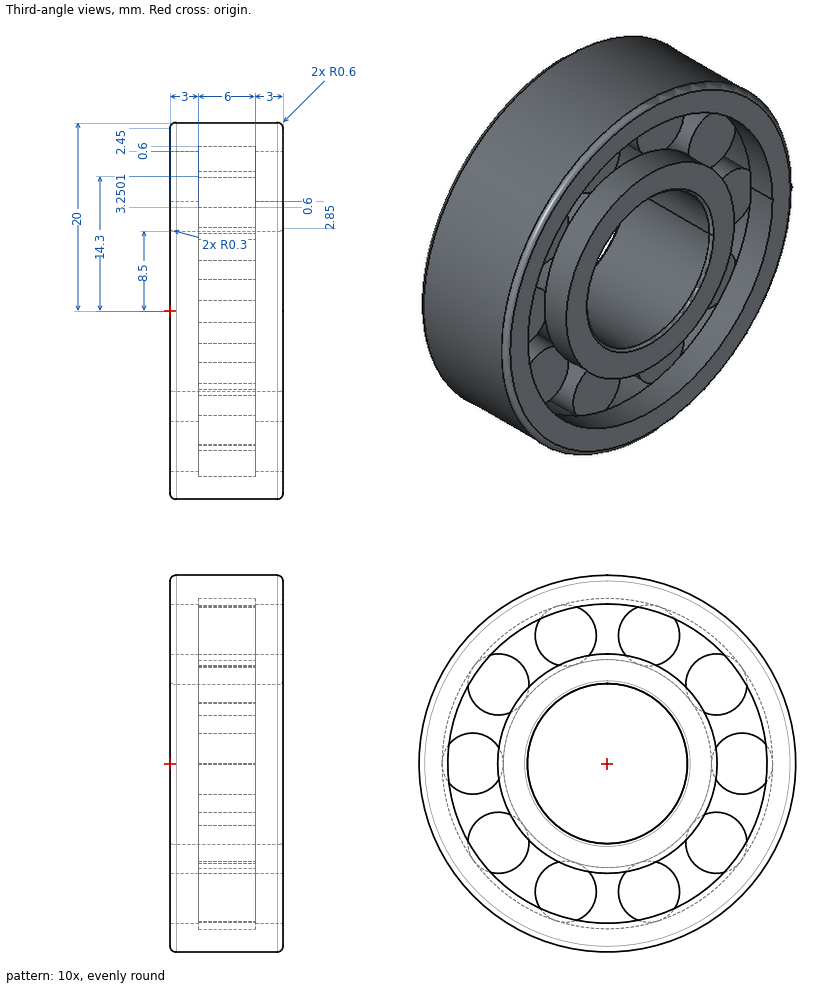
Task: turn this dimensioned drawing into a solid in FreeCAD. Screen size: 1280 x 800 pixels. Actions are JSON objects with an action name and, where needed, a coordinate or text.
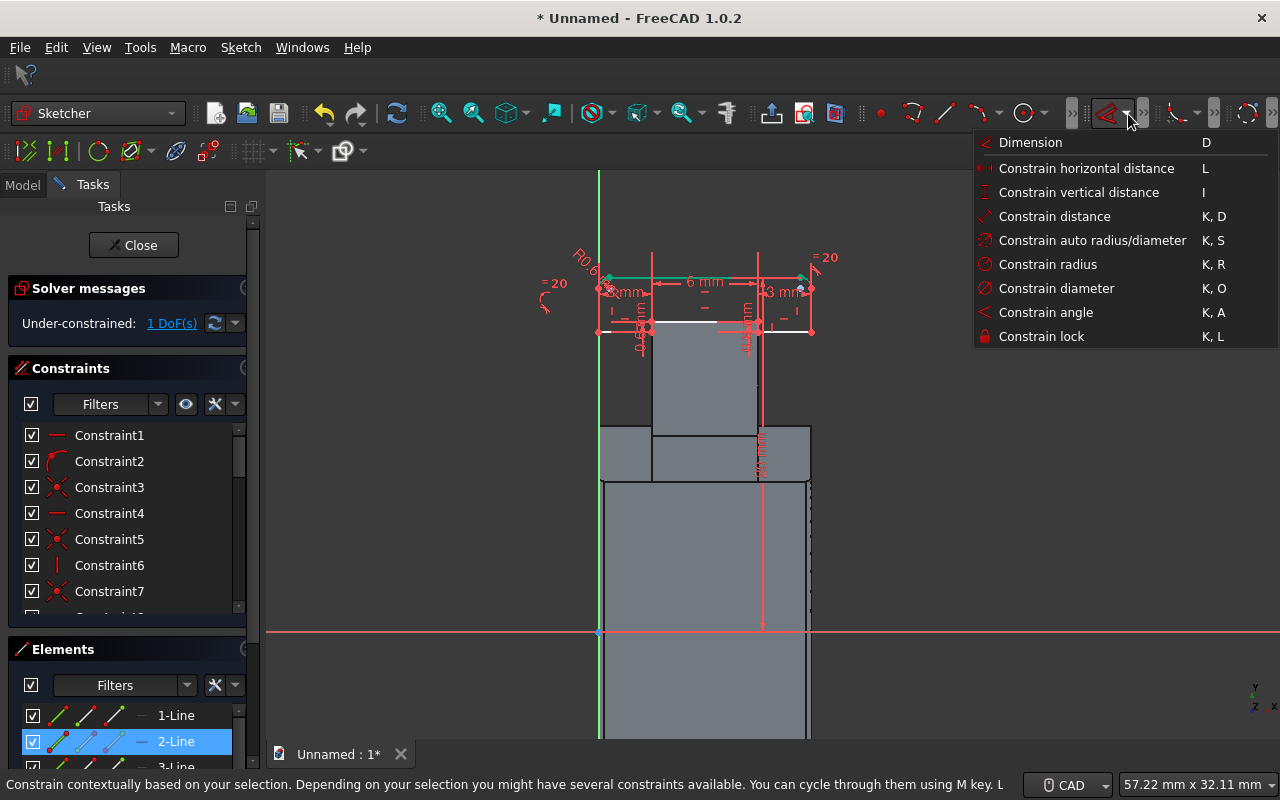
{"action": "left_click", "coordinate": [1126, 192]}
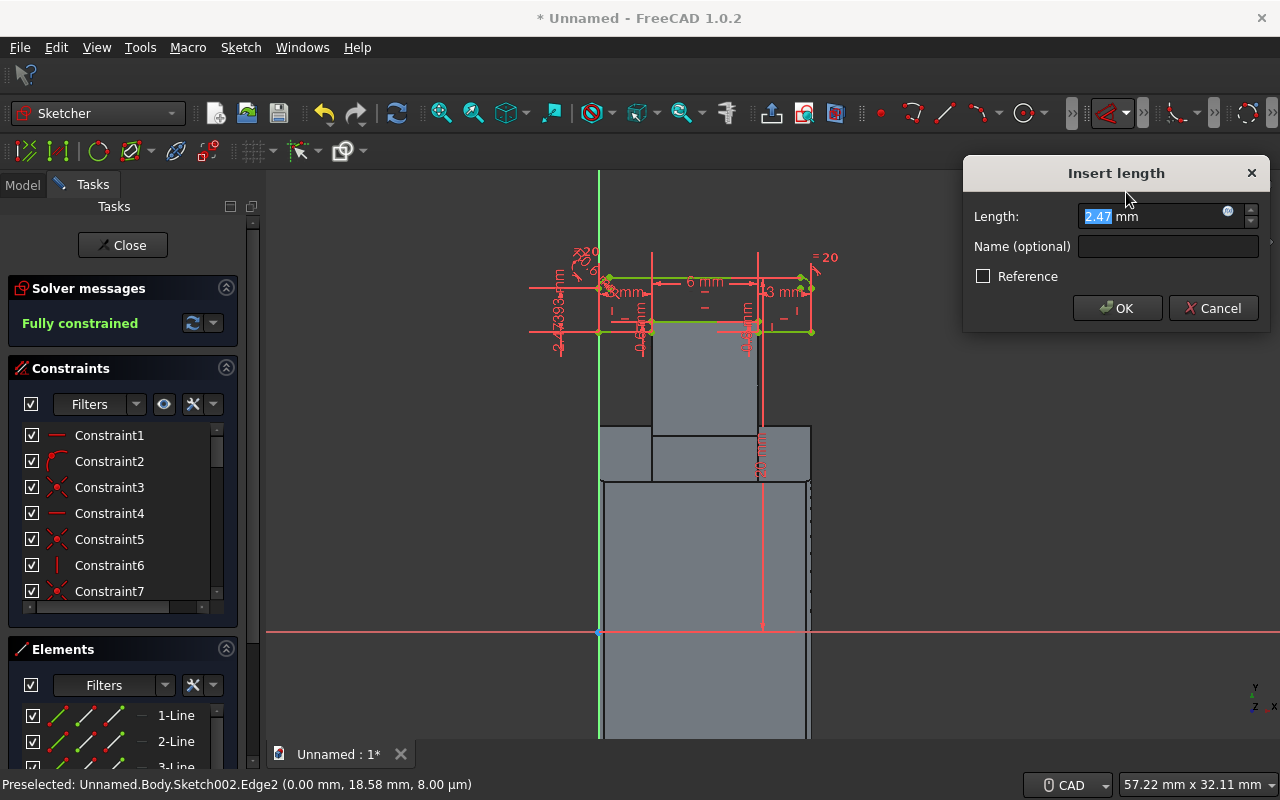
{"action": "type", "text": "2.45"}
{"action": "key", "text": "Return"}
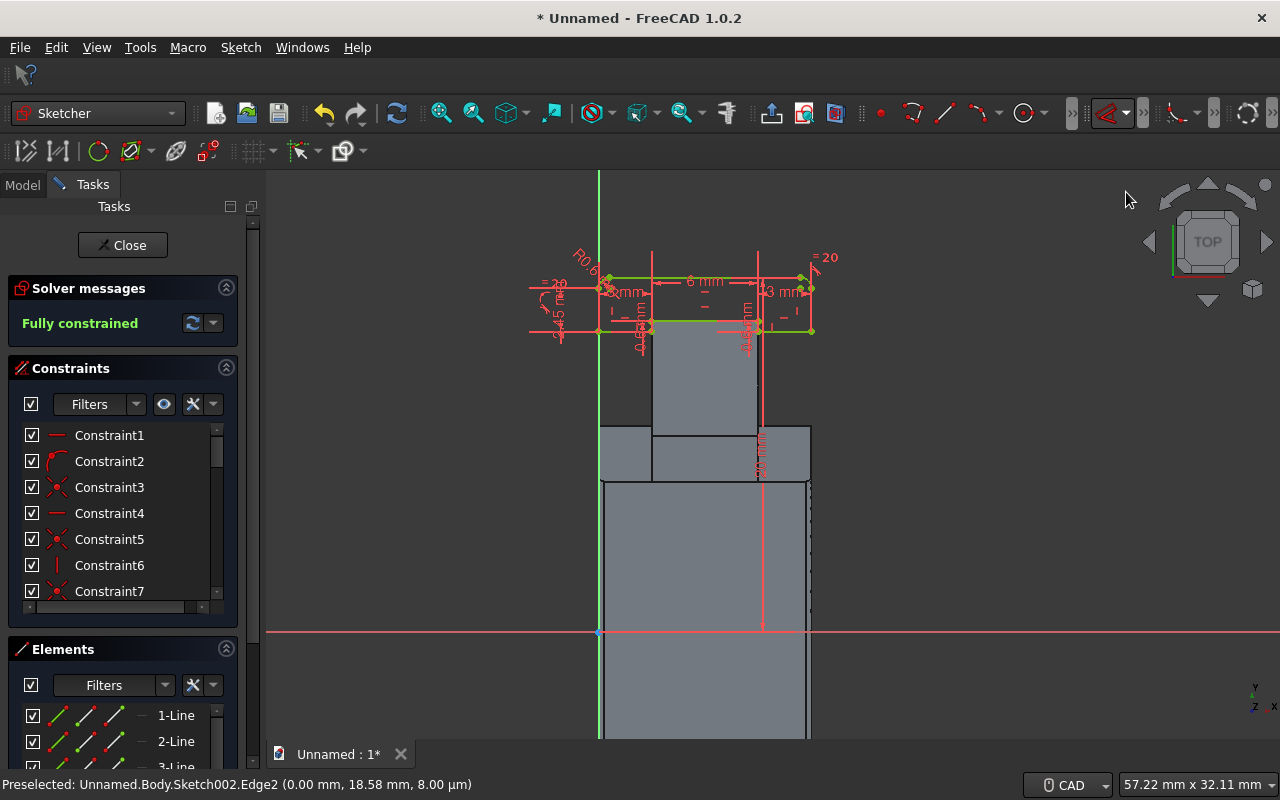
{"action": "left_click", "coordinate": [123, 245]}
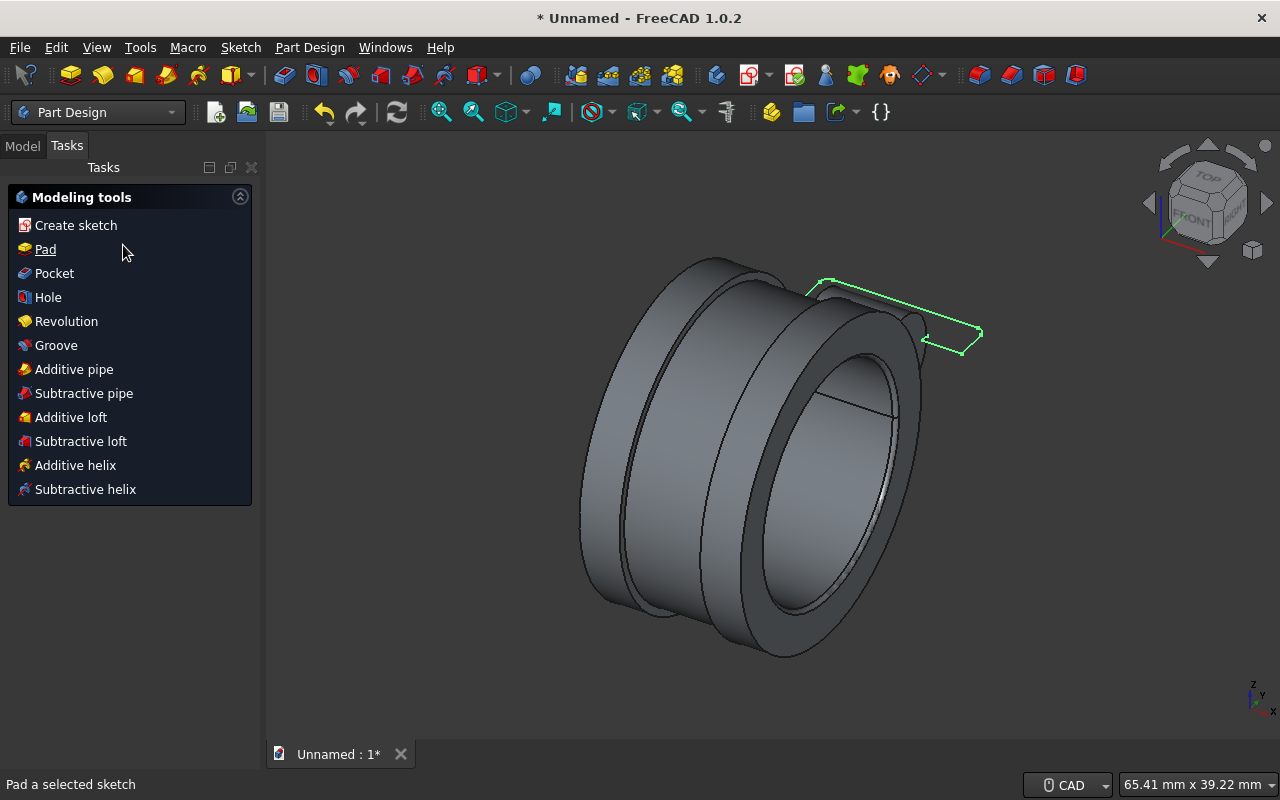
{"action": "left_click", "coordinate": [104, 76]}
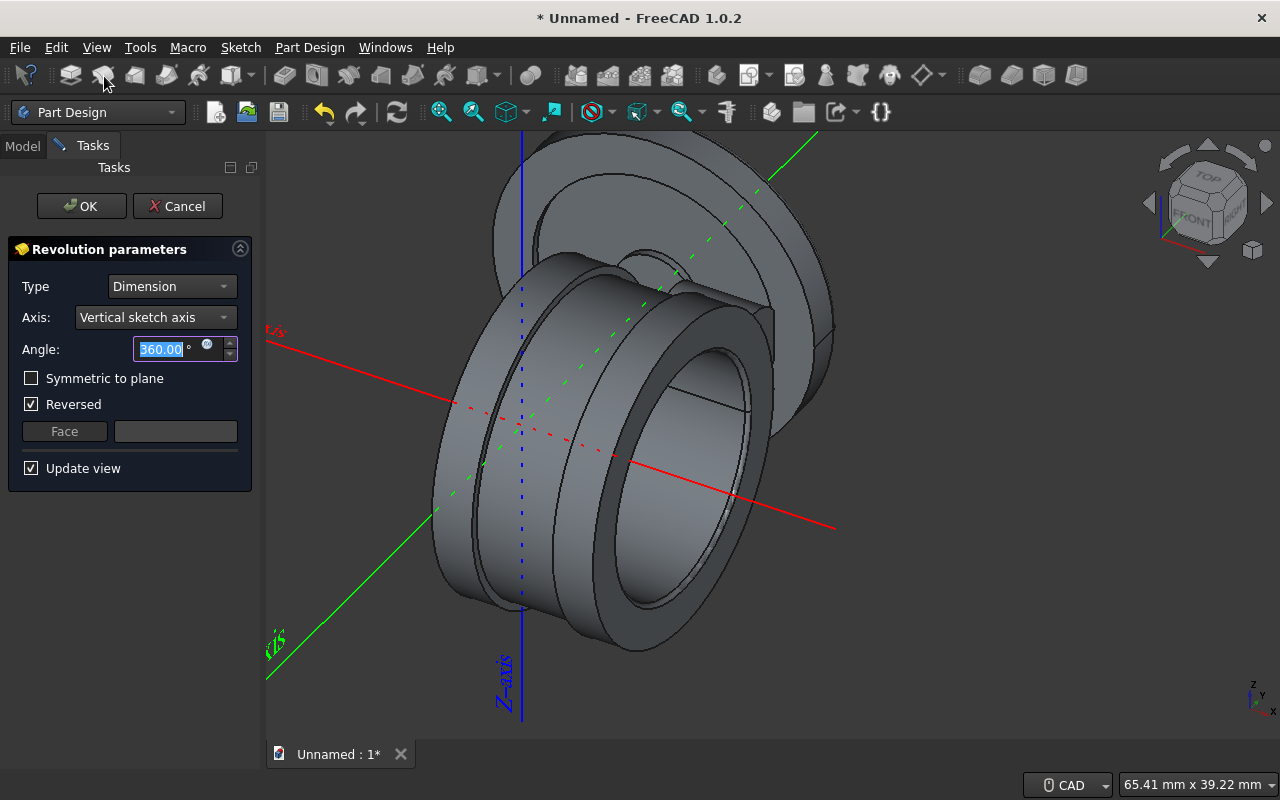
{"action": "left_click", "coordinate": [156, 318]}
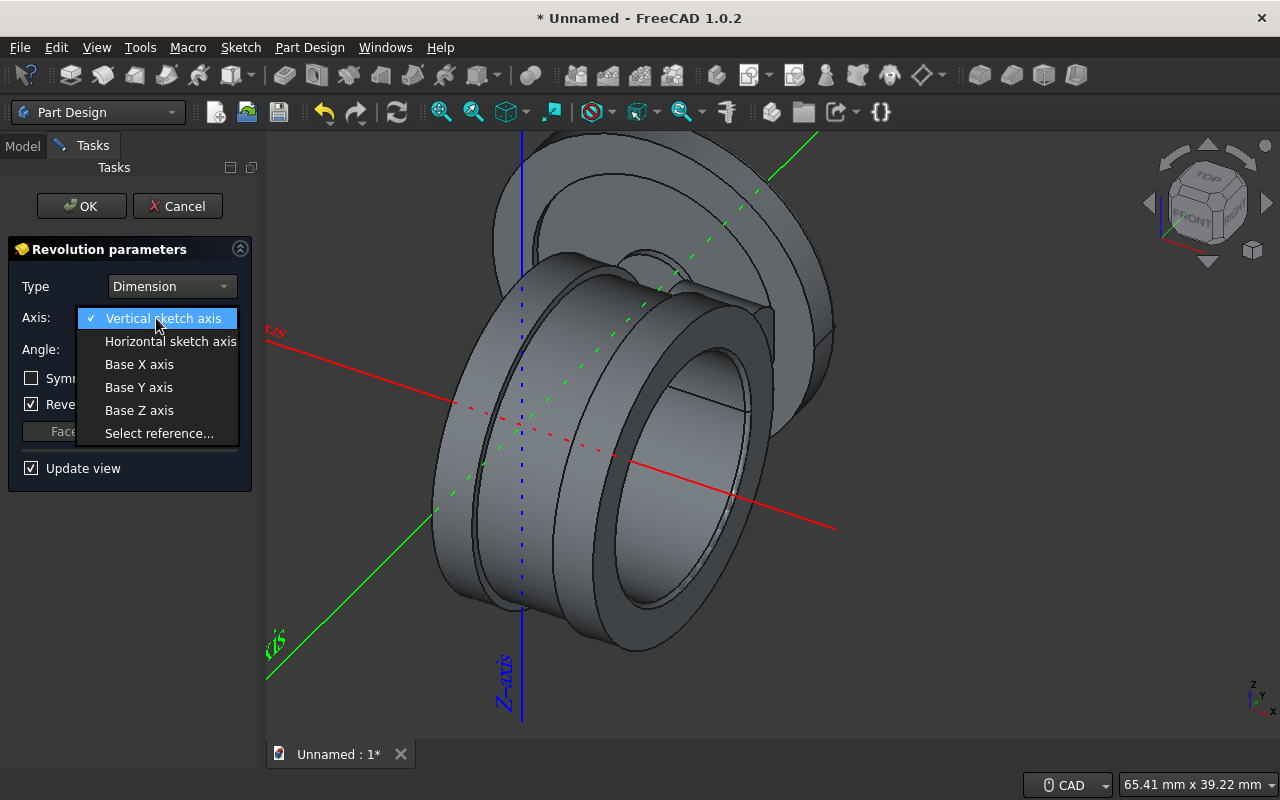
{"action": "left_click", "coordinate": [156, 342]}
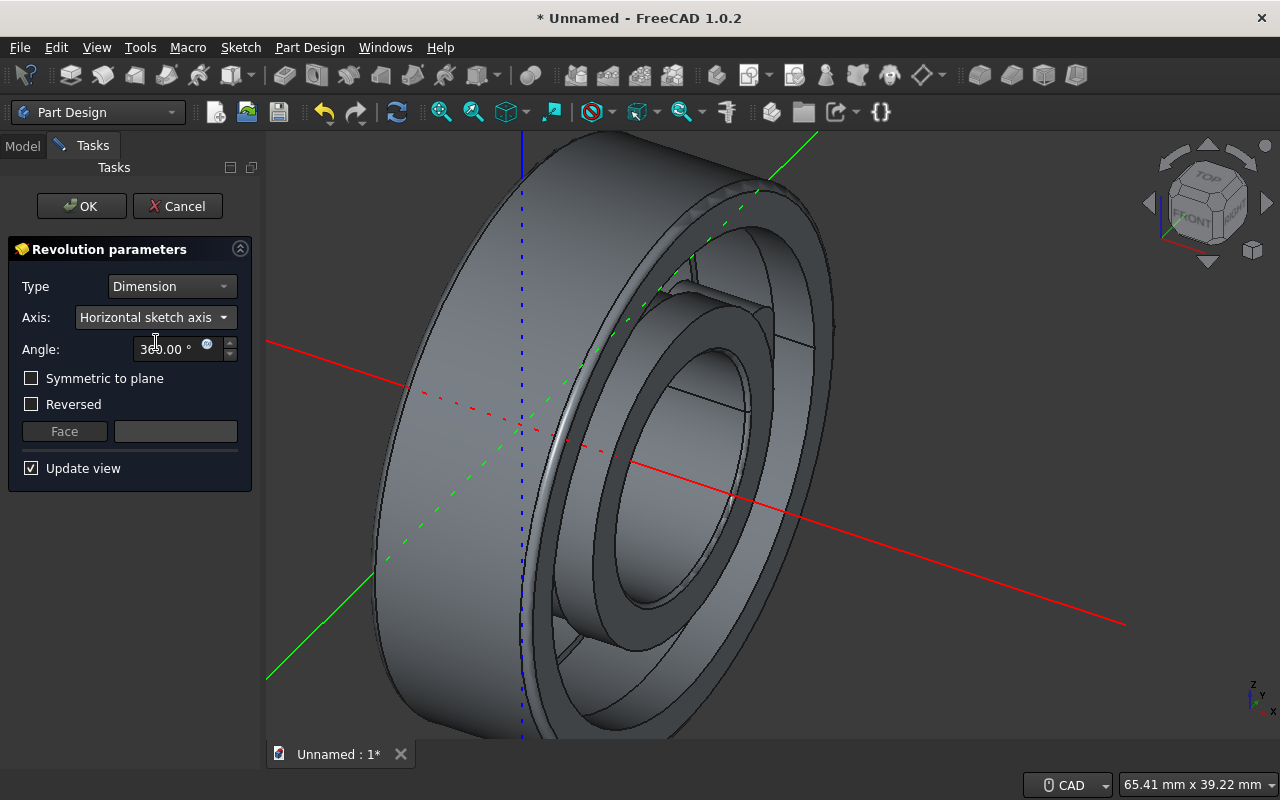
{"action": "left_click", "coordinate": [82, 206]}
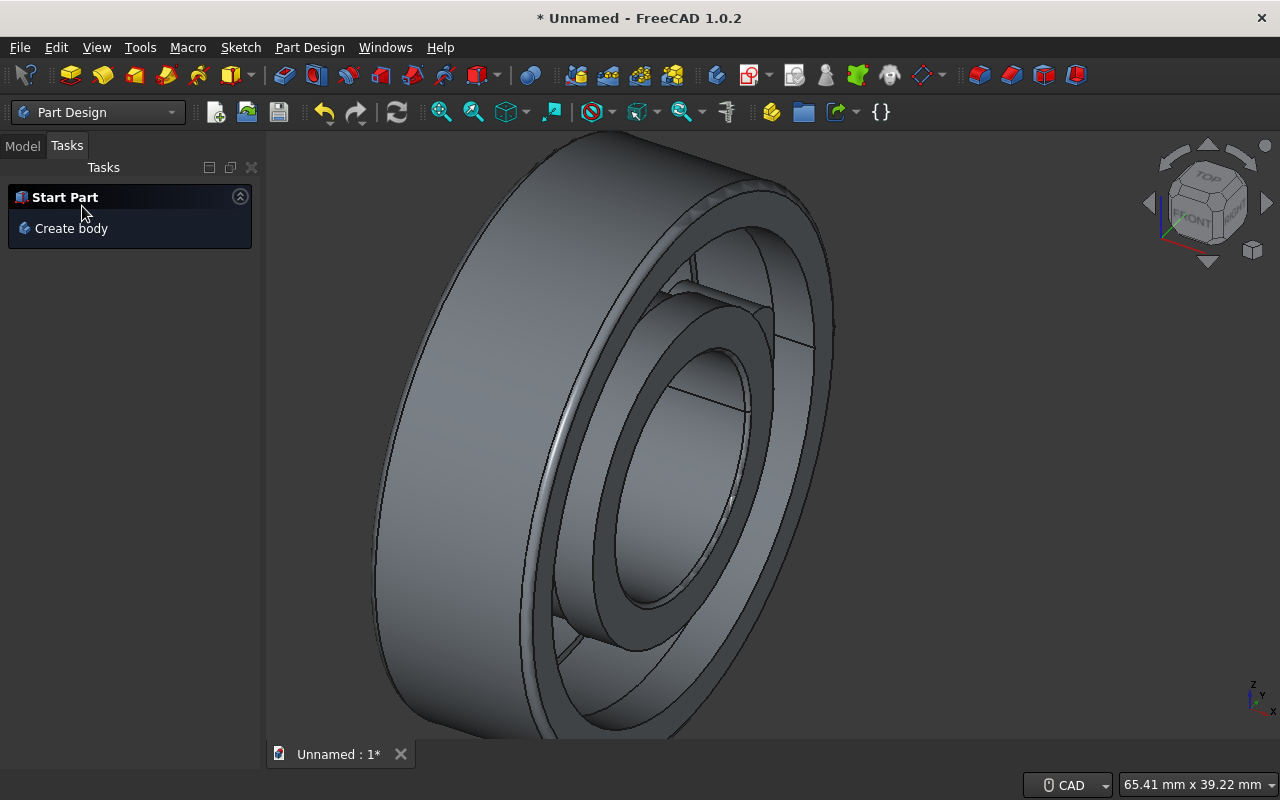
{"action": "left_click", "coordinate": [442, 112]}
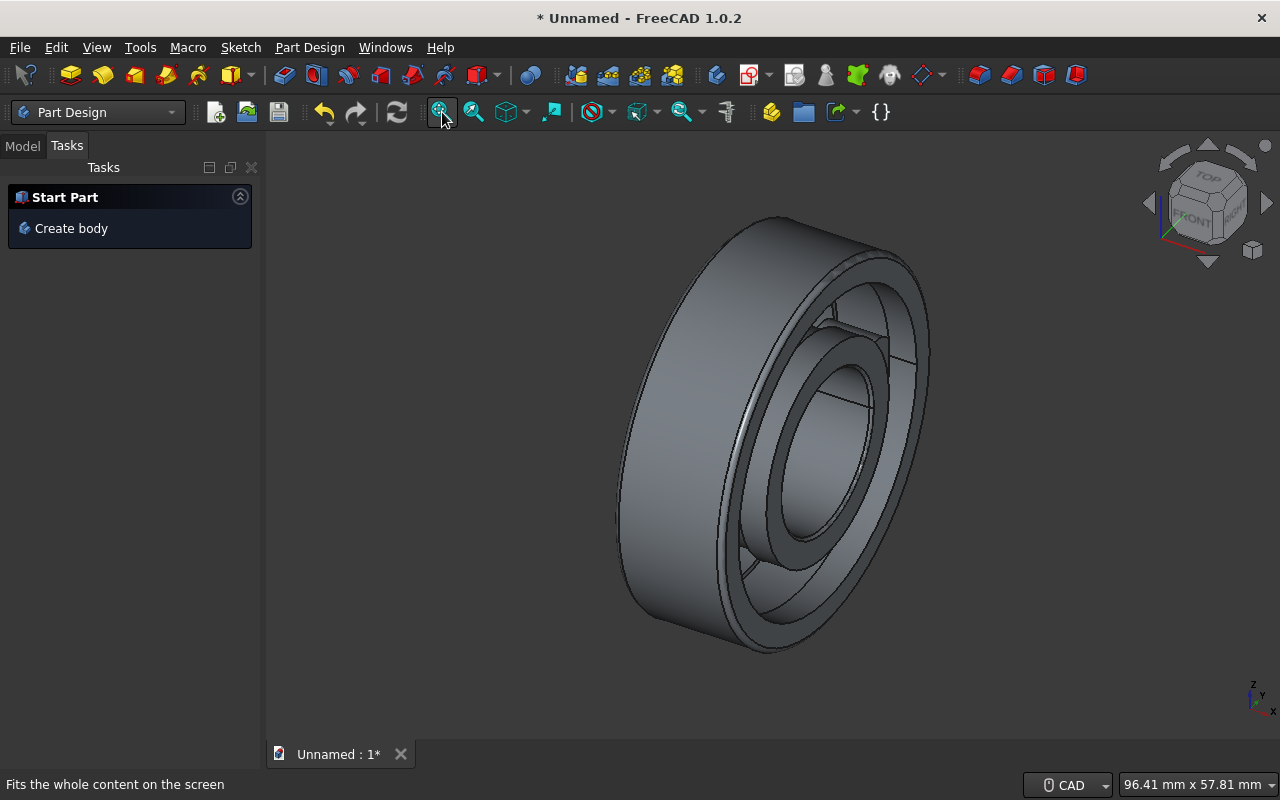
{"action": "left_click", "coordinate": [23, 145]}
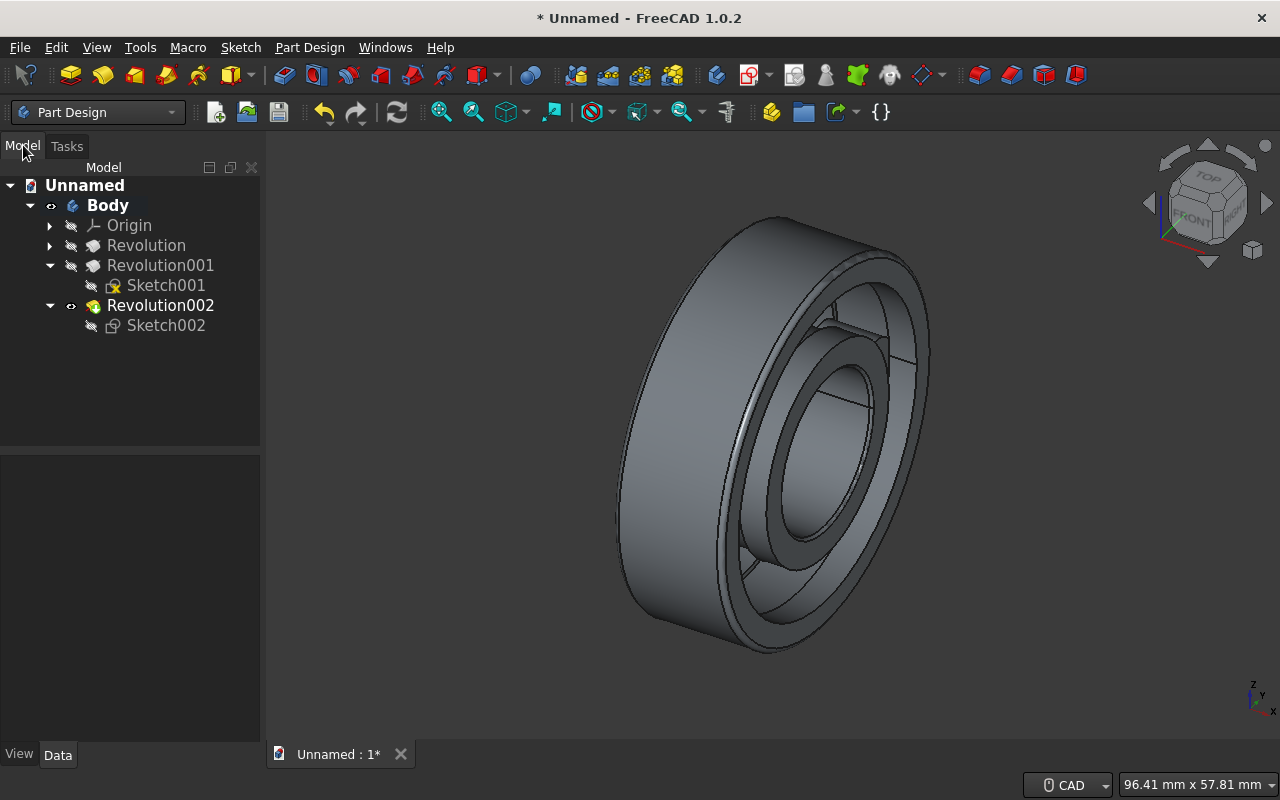
{"action": "left_click", "coordinate": [116, 266]}